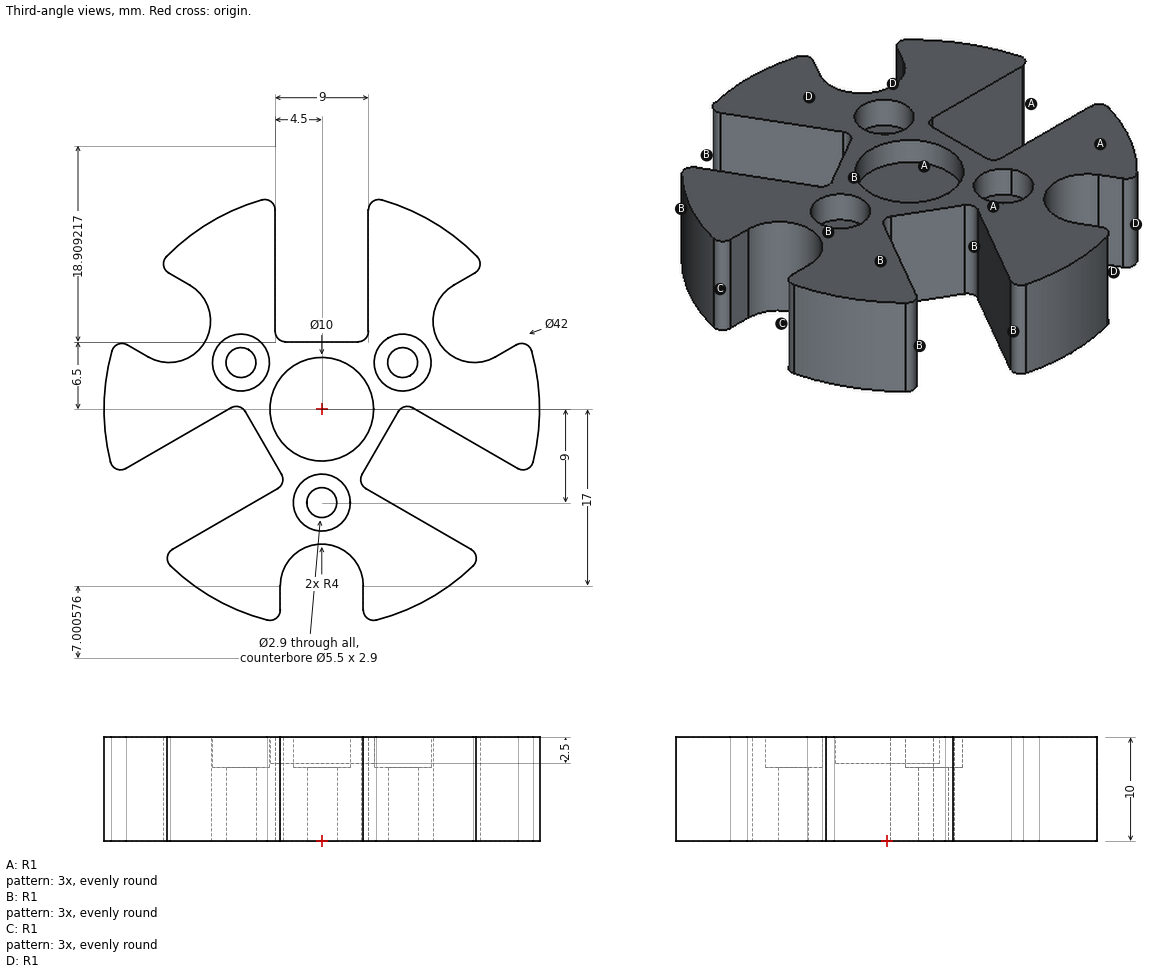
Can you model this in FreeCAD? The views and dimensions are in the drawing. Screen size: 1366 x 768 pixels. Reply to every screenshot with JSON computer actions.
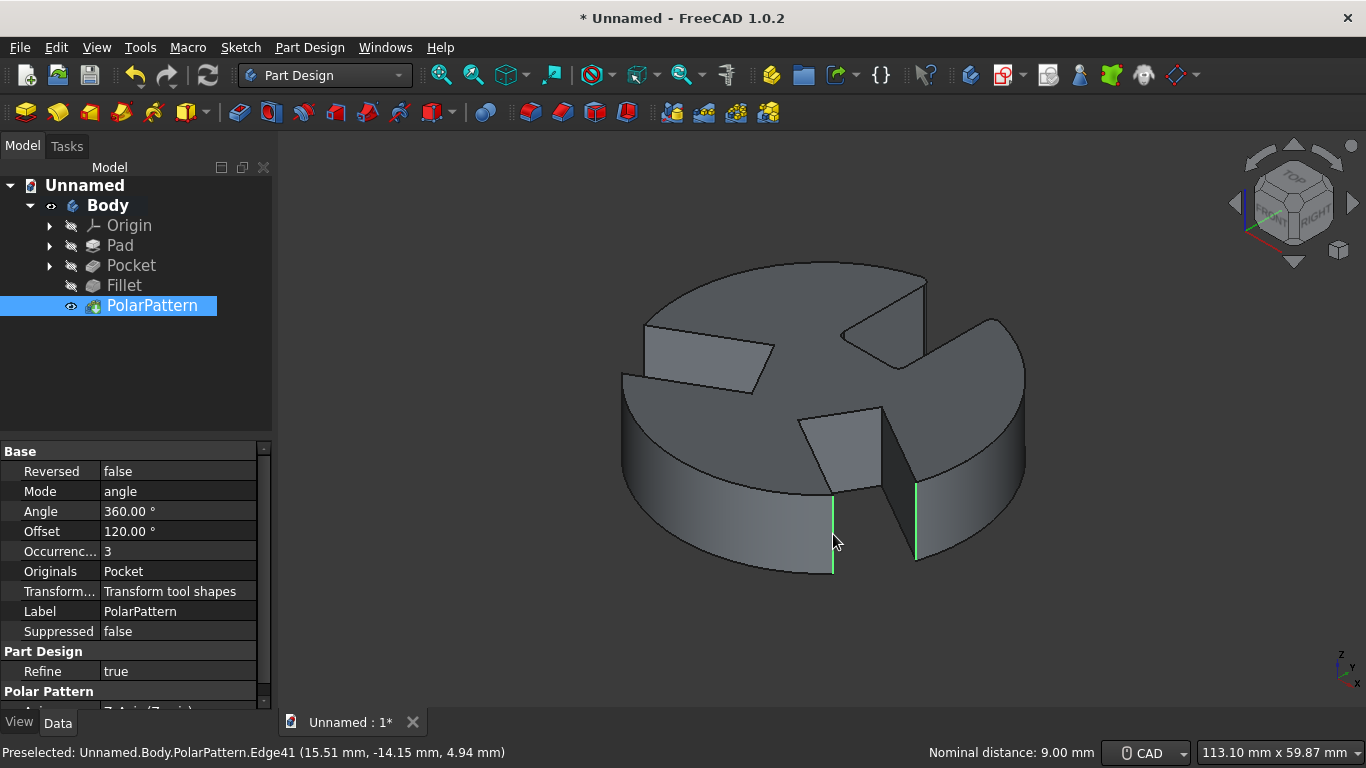
{"action": "key", "text": "2"}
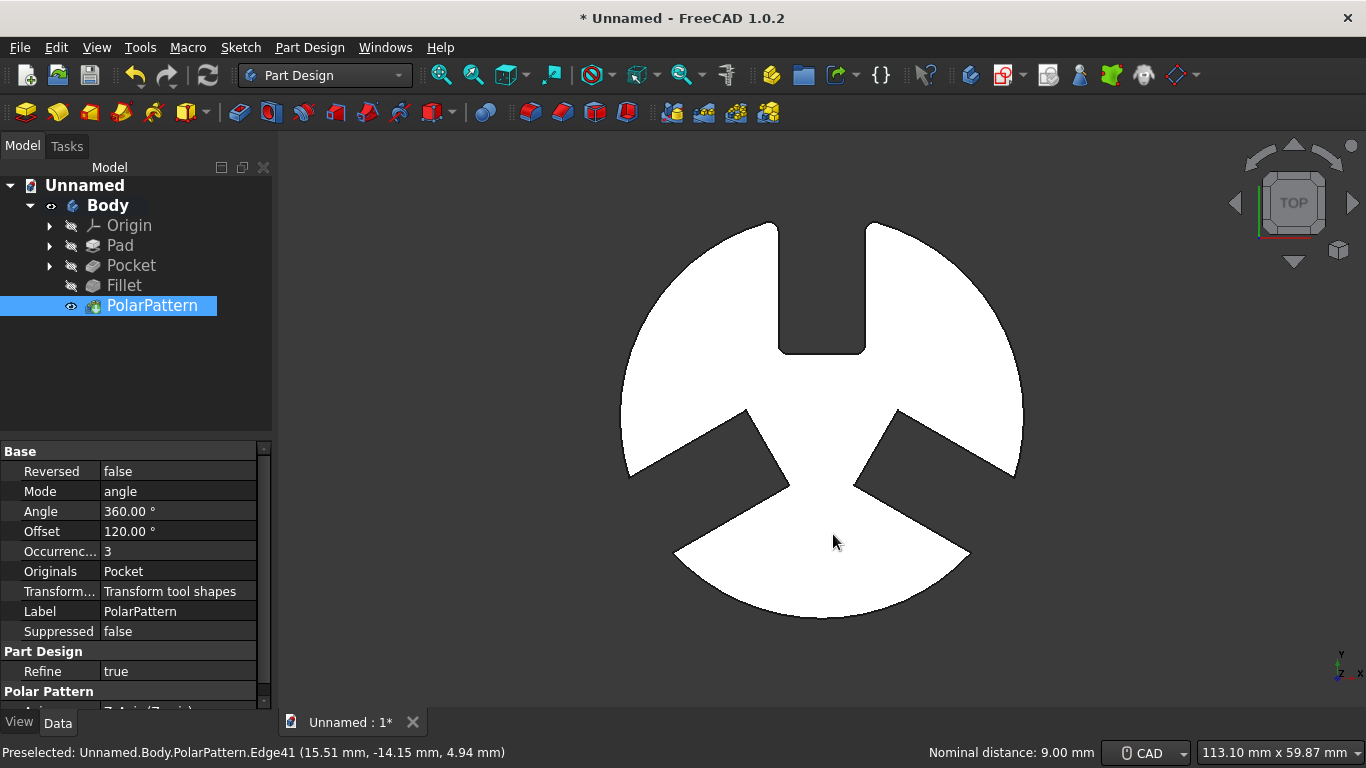
{"action": "key", "text": "0"}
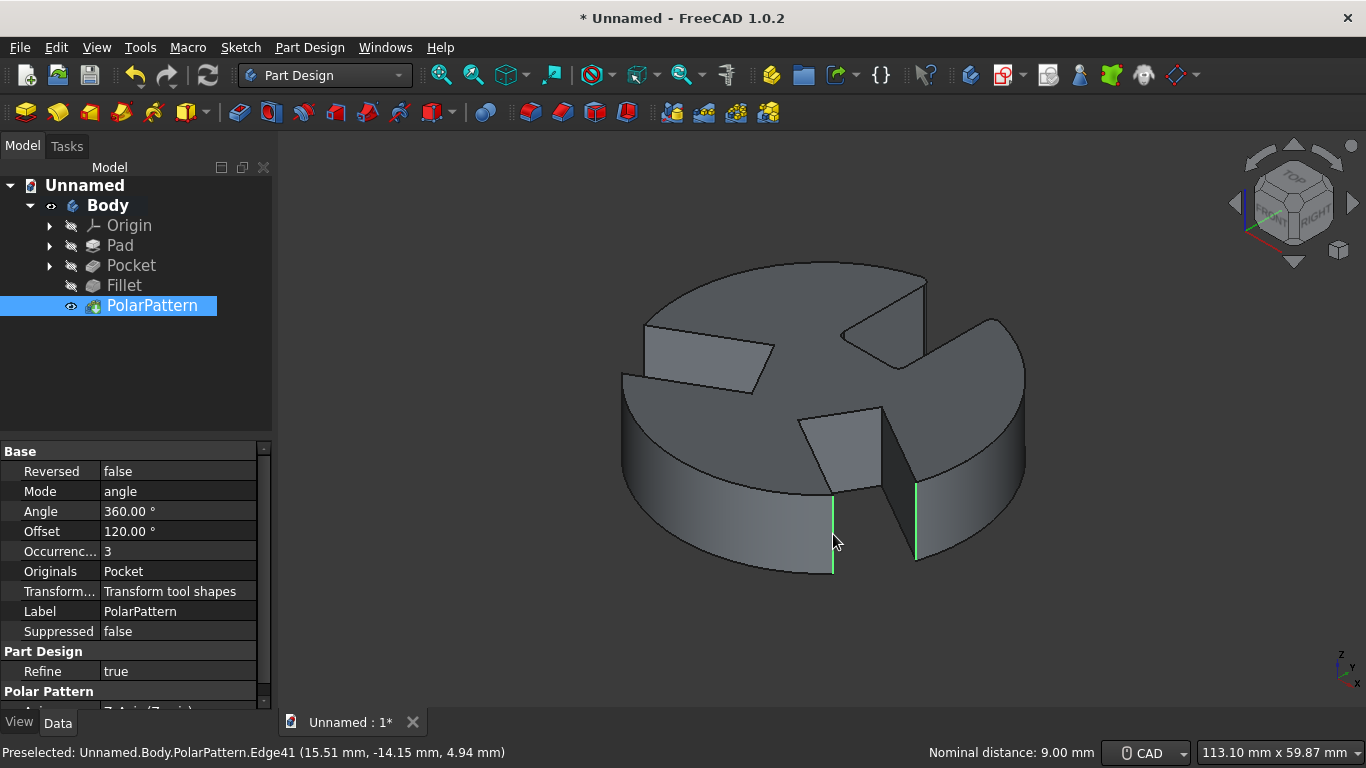
{"action": "key", "text": "1"}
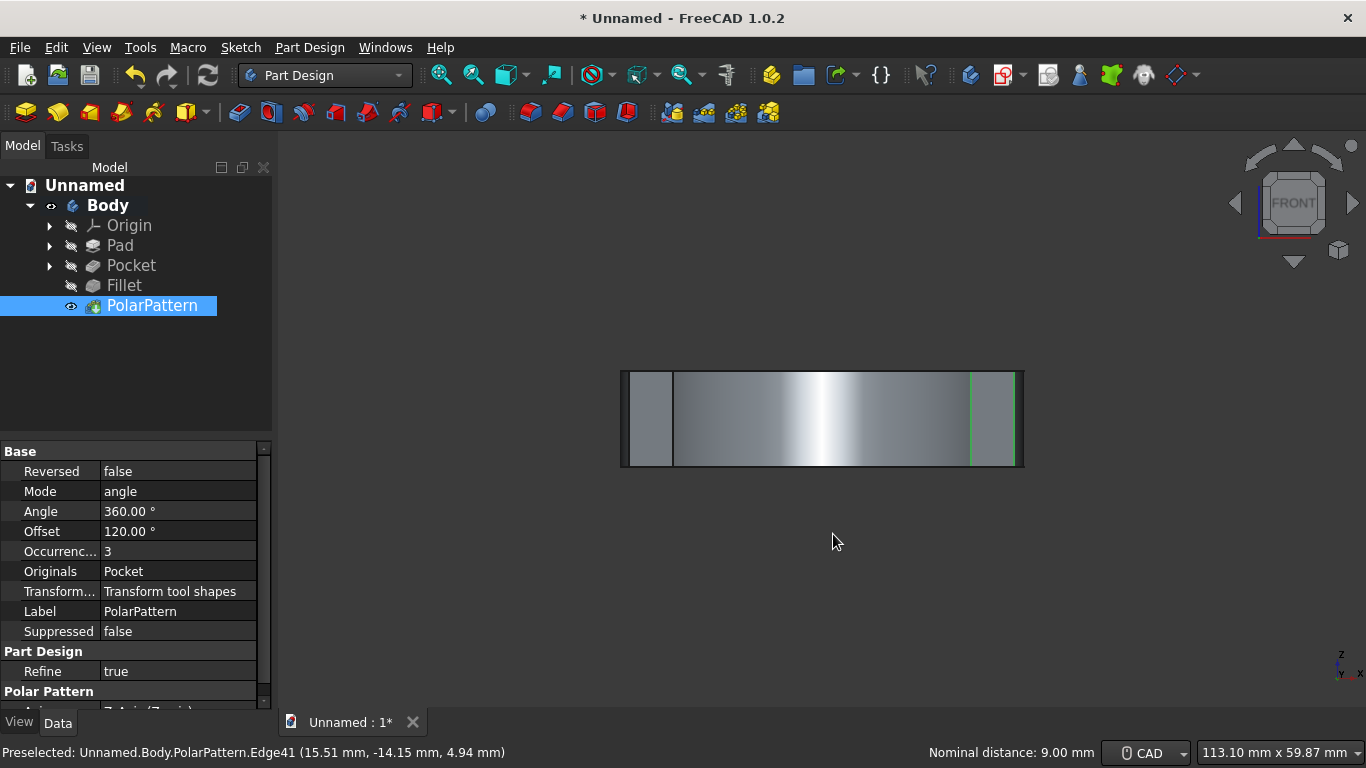
{"action": "left_click", "coordinate": [442, 76]}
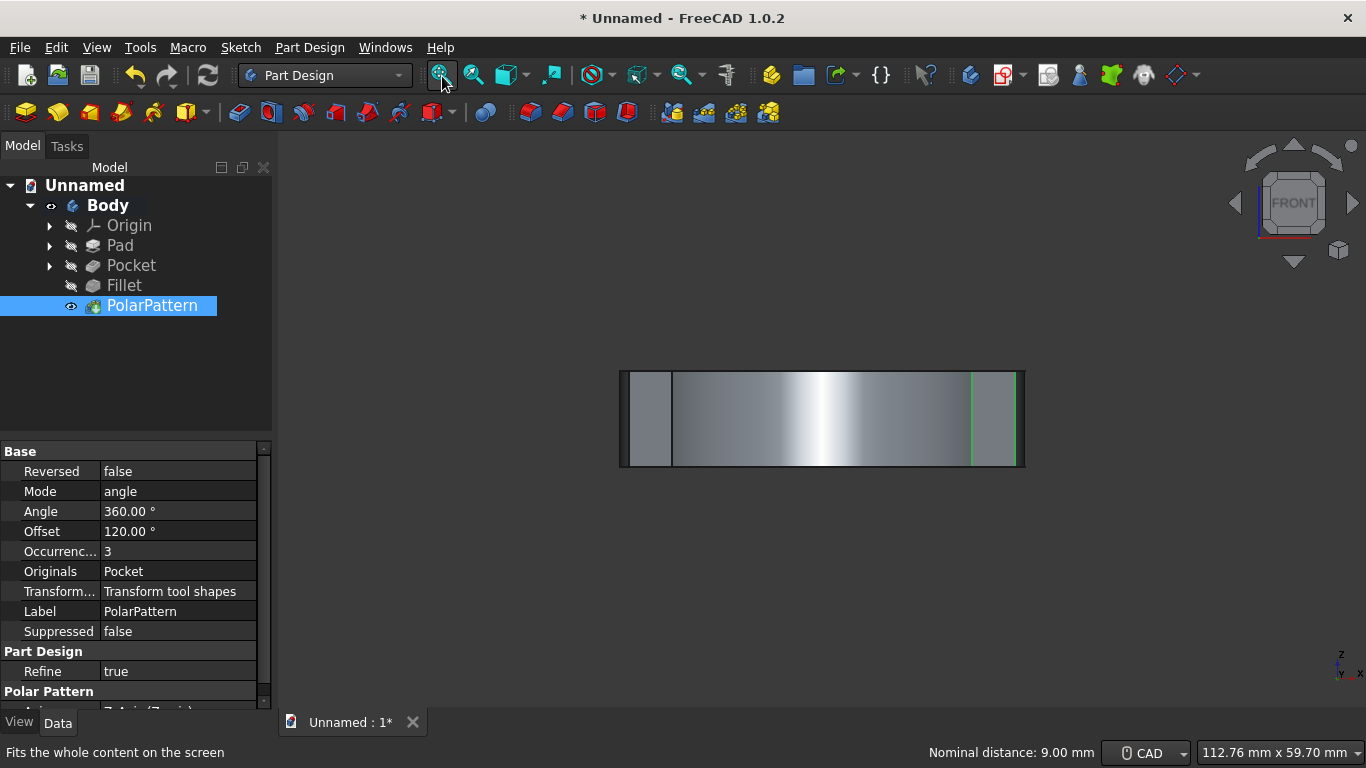
{"action": "left_click", "coordinate": [629, 418], "text": "ctrl"}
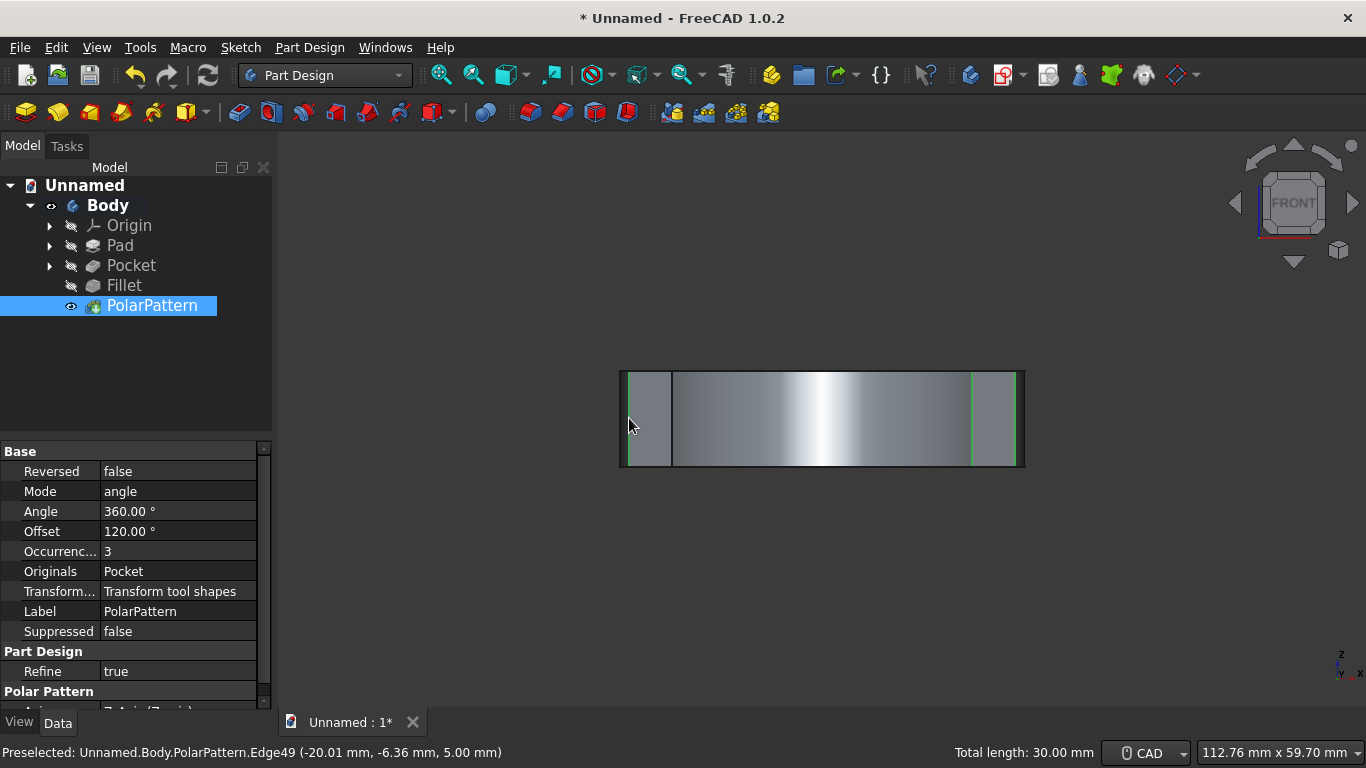
{"action": "key", "text": "3"}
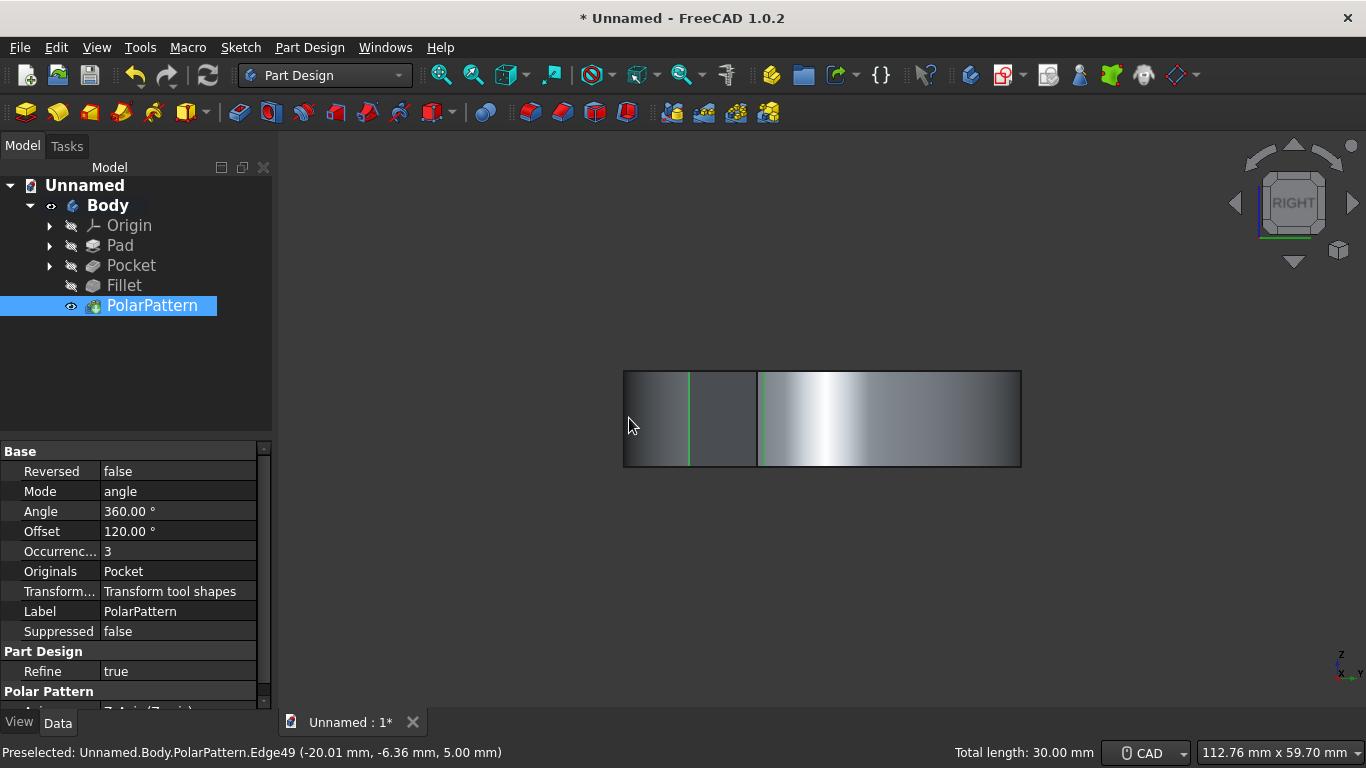
{"action": "left_click", "coordinate": [442, 76]}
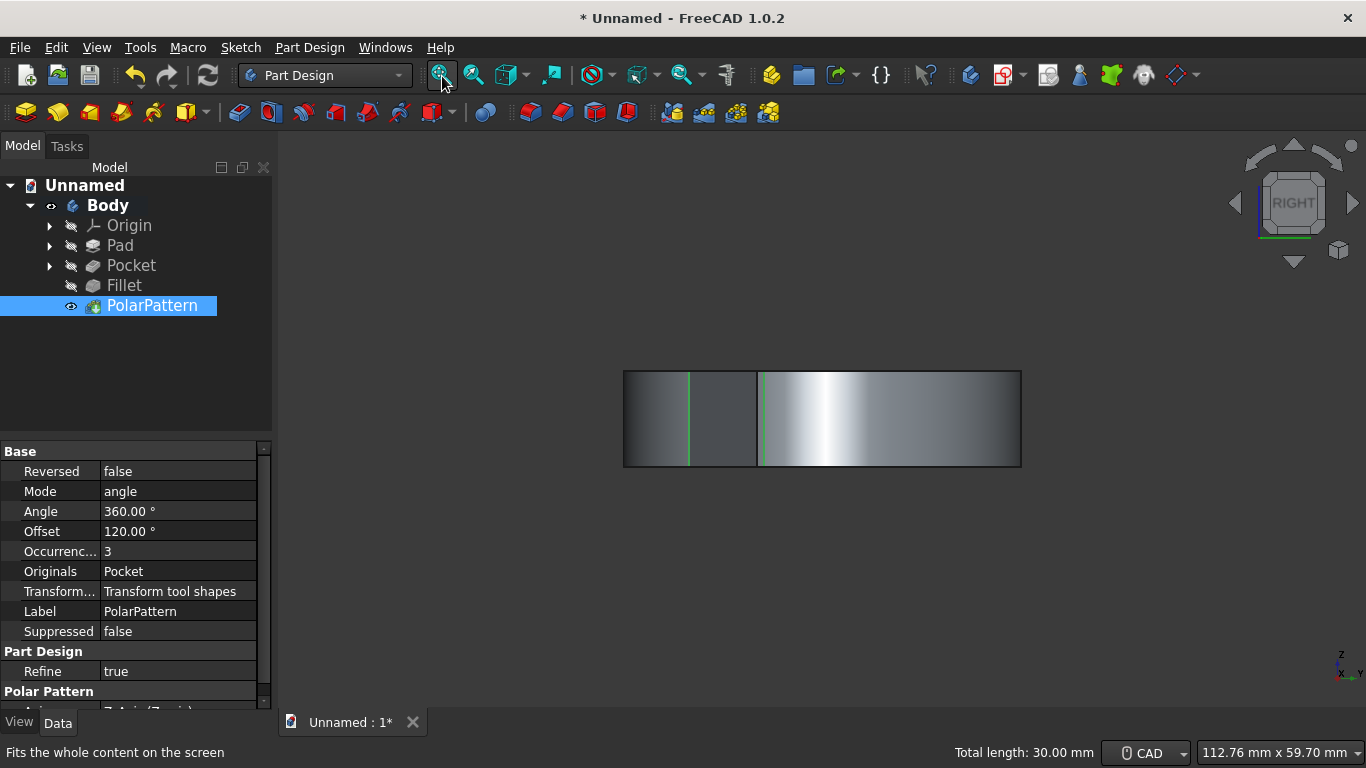
{"action": "key", "text": "5"}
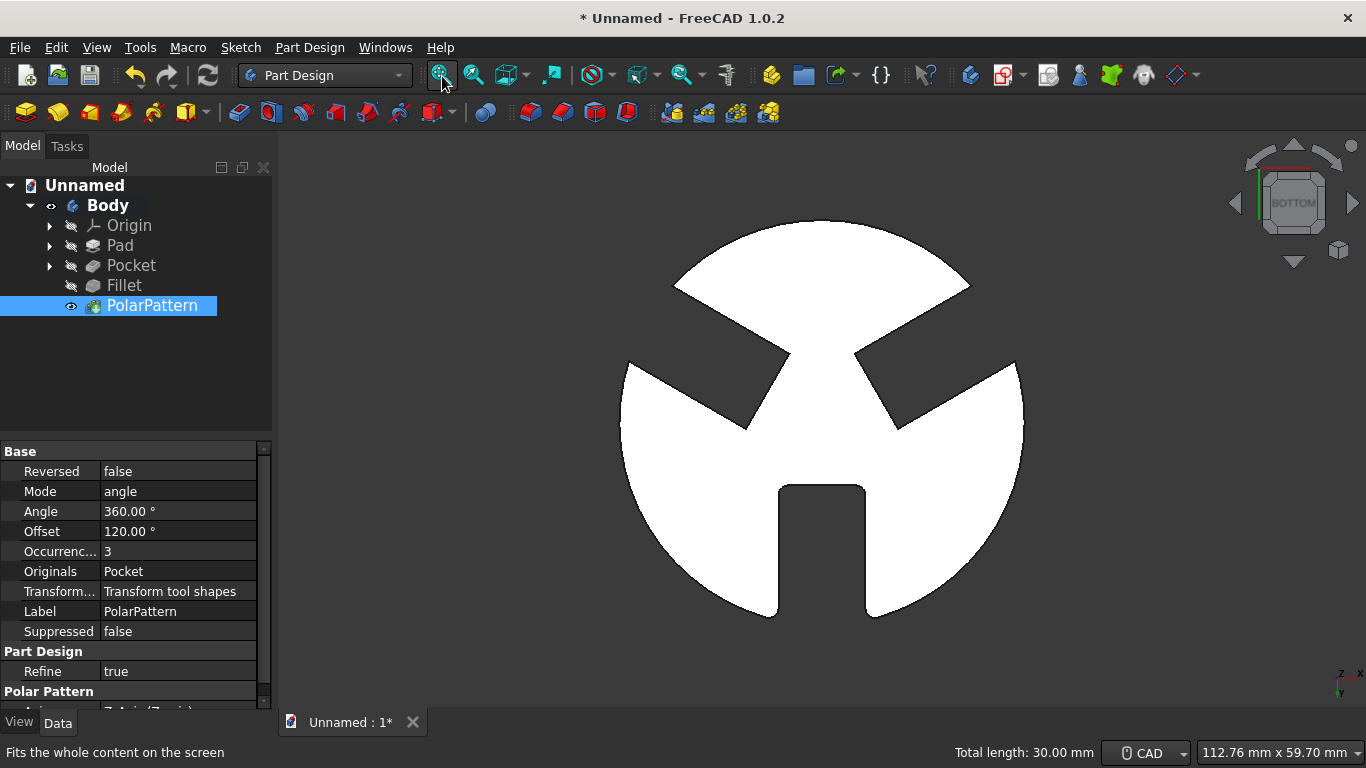
{"action": "key", "text": "4"}